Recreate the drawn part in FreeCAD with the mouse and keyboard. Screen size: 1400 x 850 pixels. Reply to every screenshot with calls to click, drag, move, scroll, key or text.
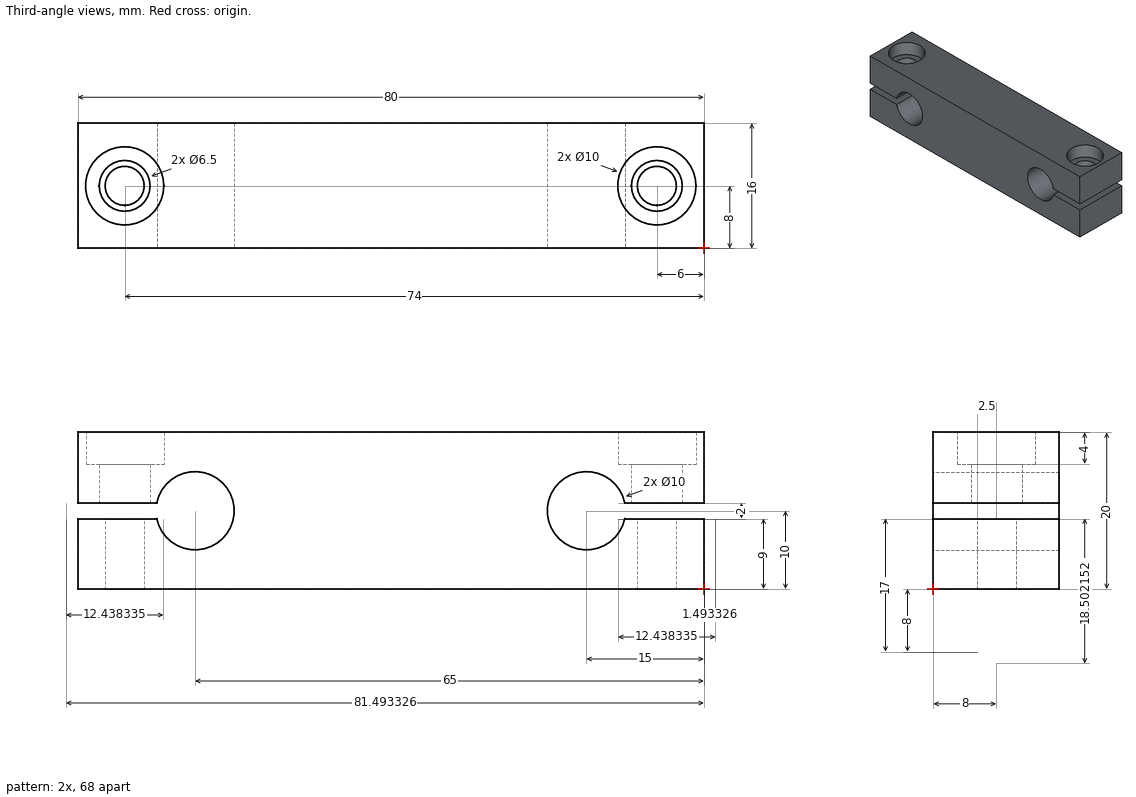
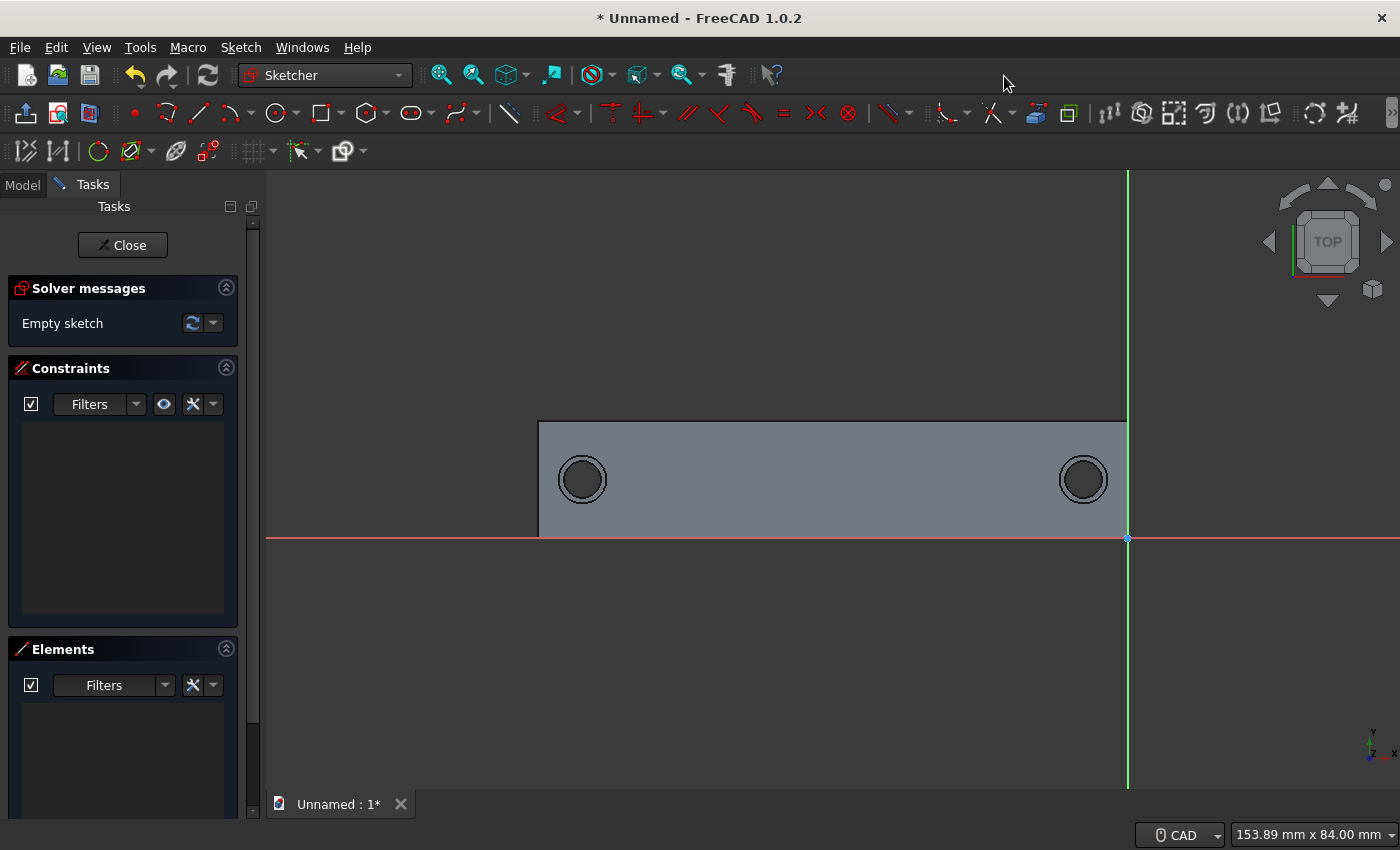
click(276, 114)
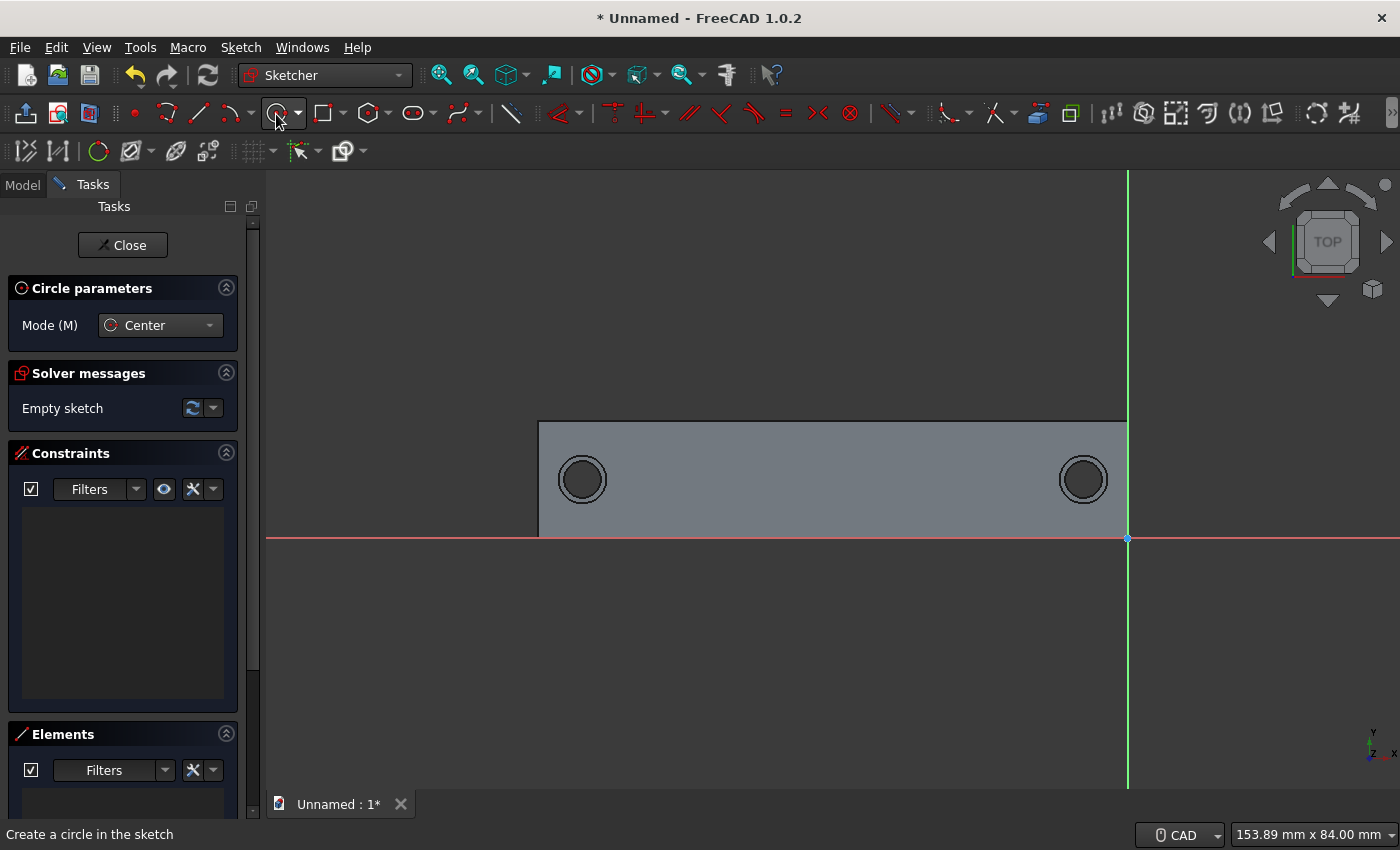
click(1084, 480)
click(1110, 453)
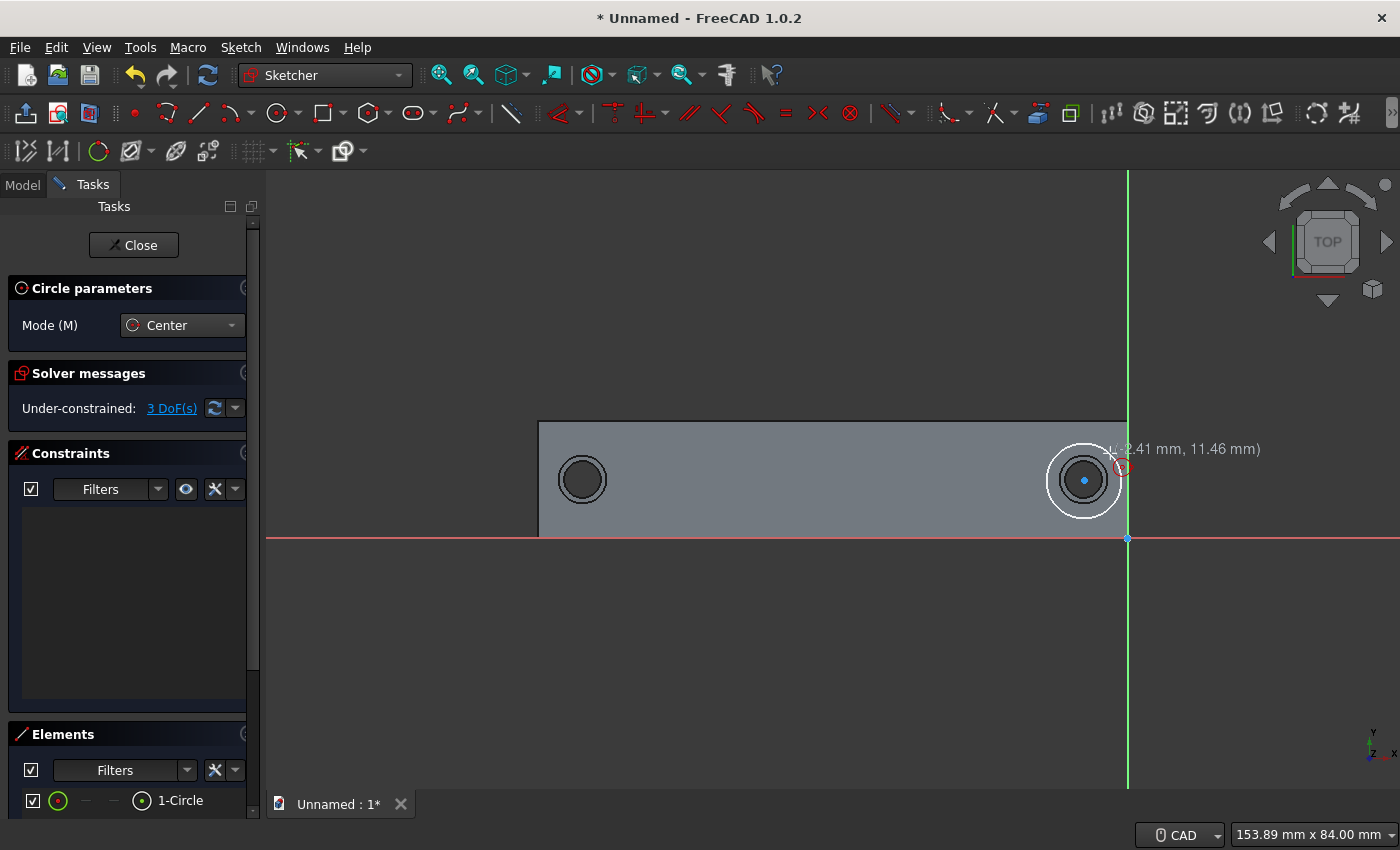
click(582, 480)
click(609, 453)
key(Escape)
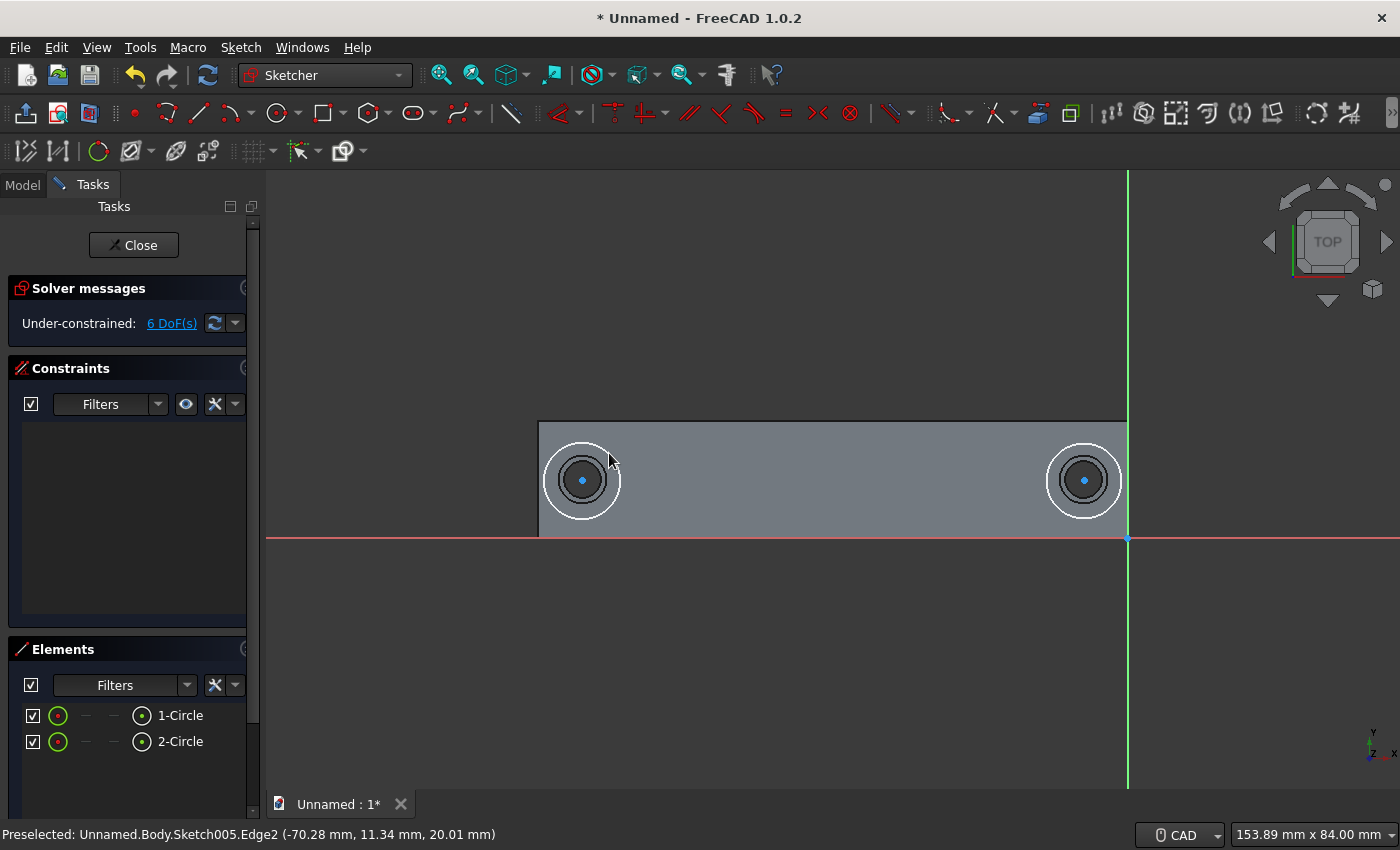
click(1110, 454)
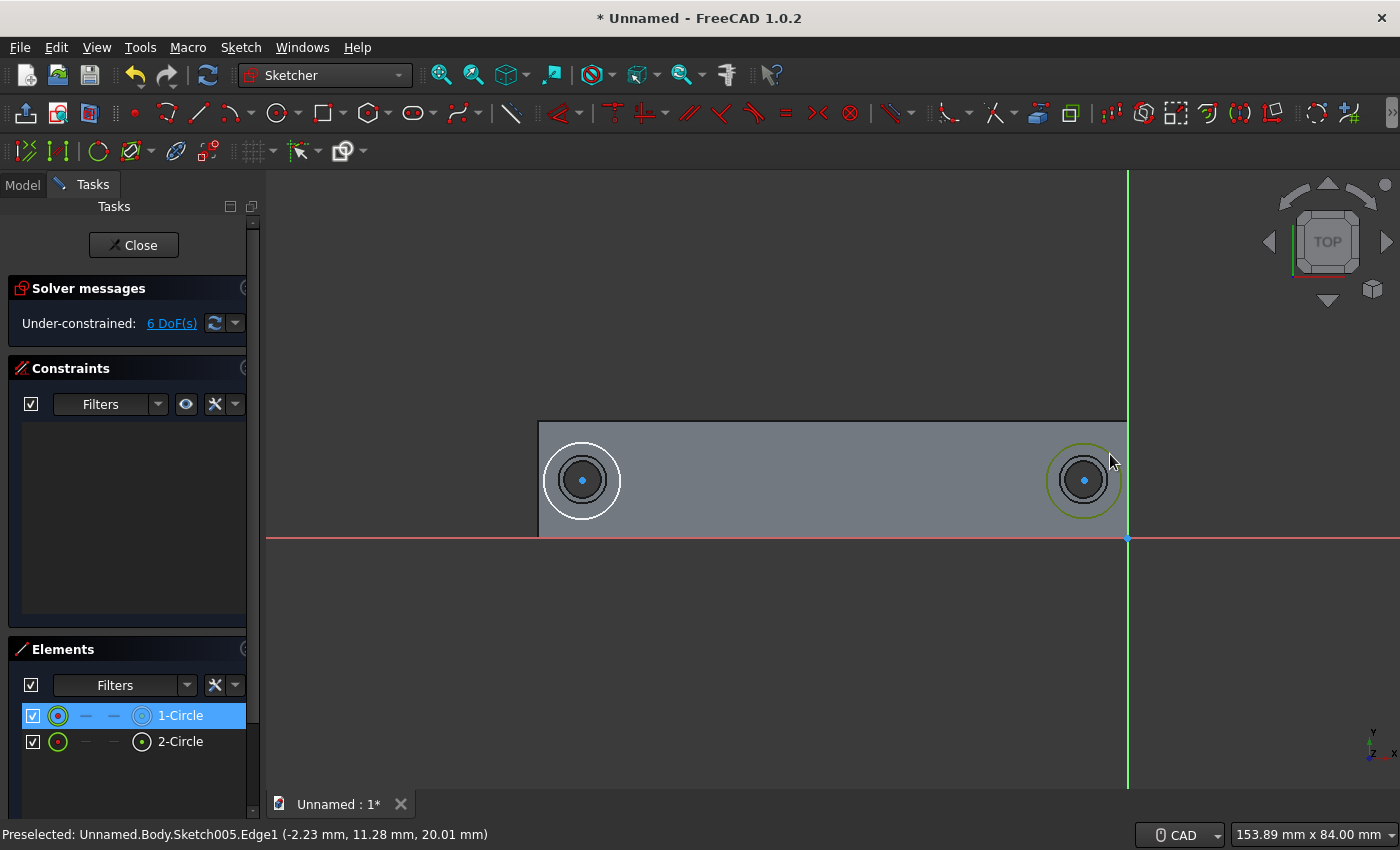
click(609, 454)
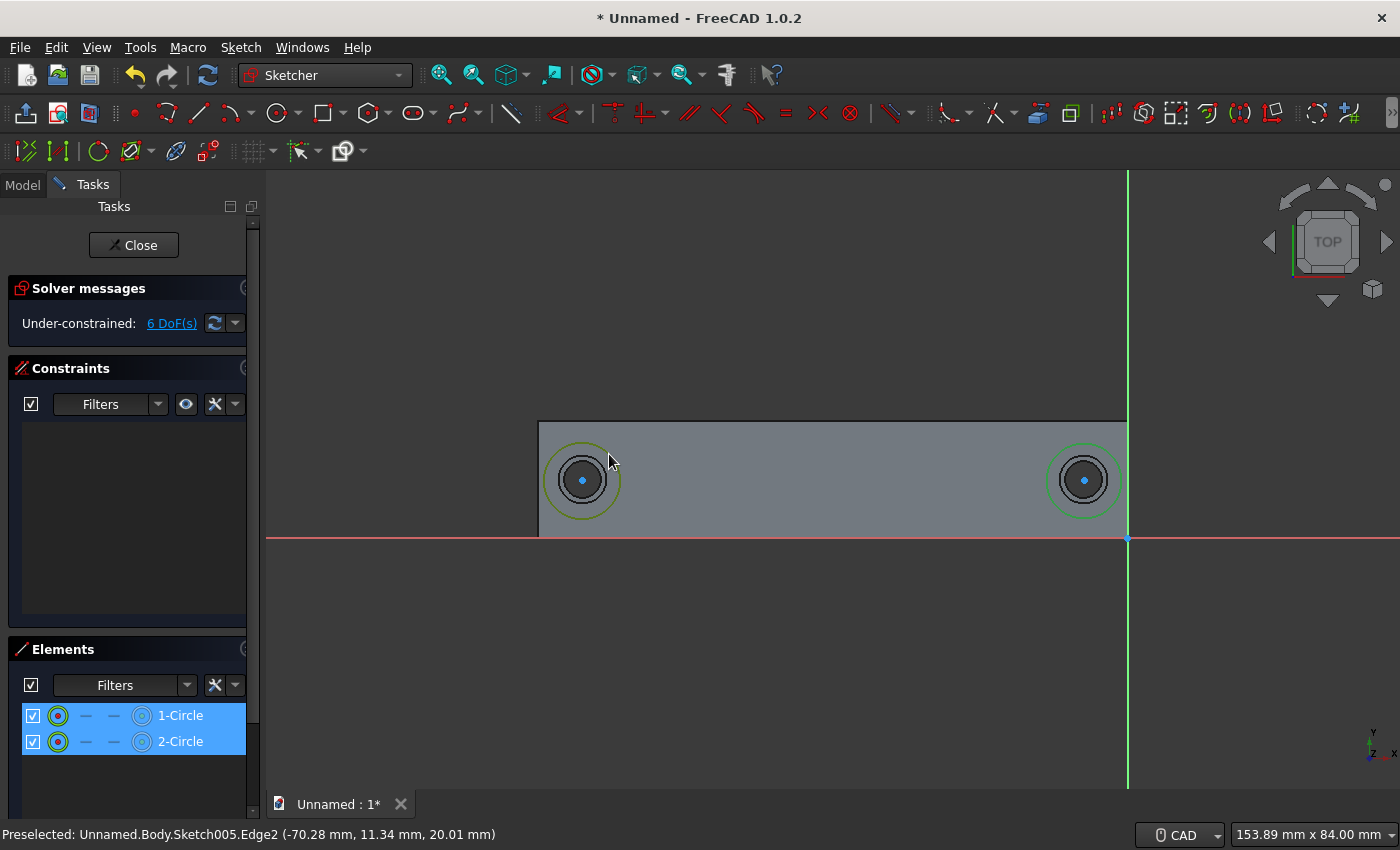
click(786, 114)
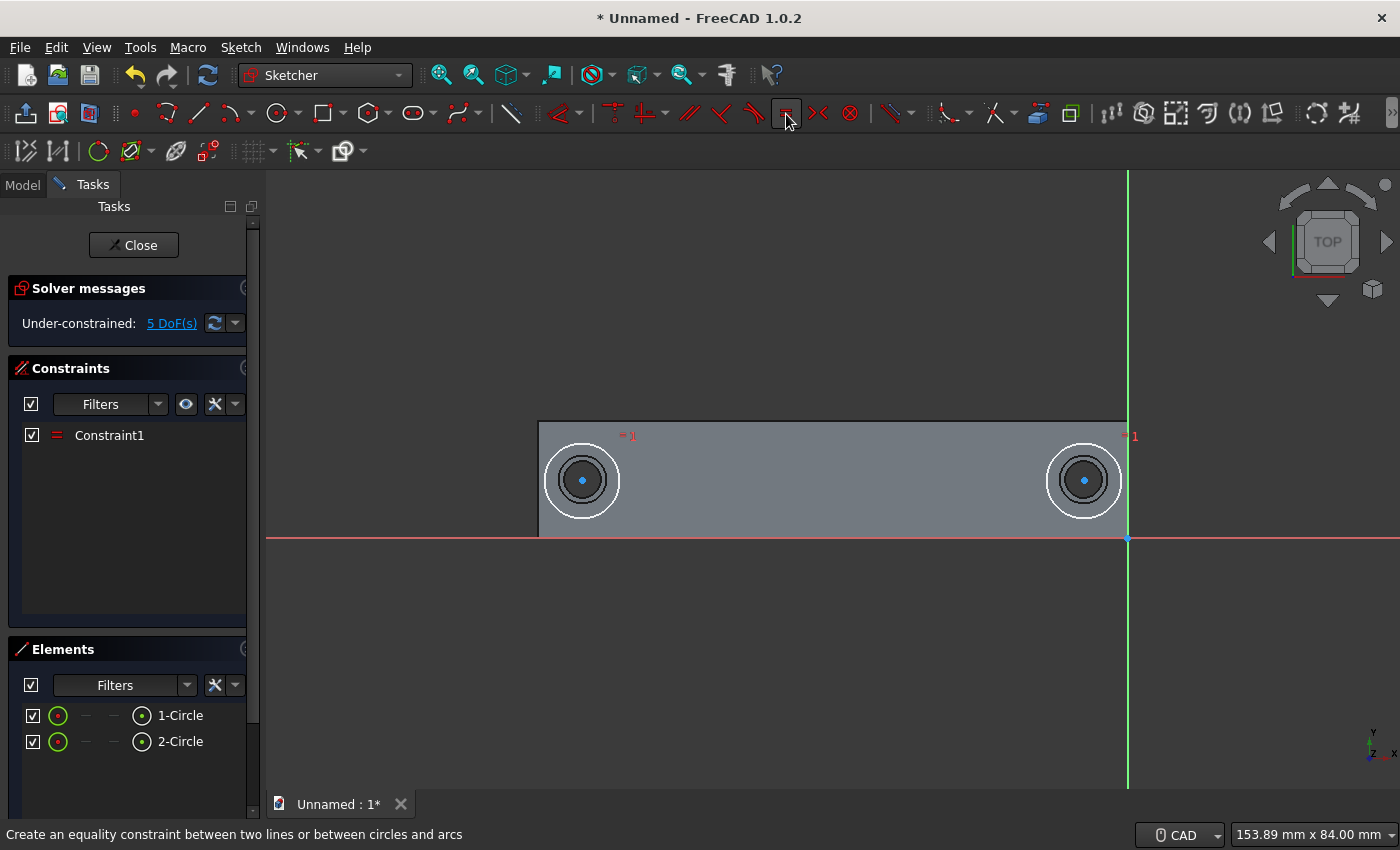
click(558, 114)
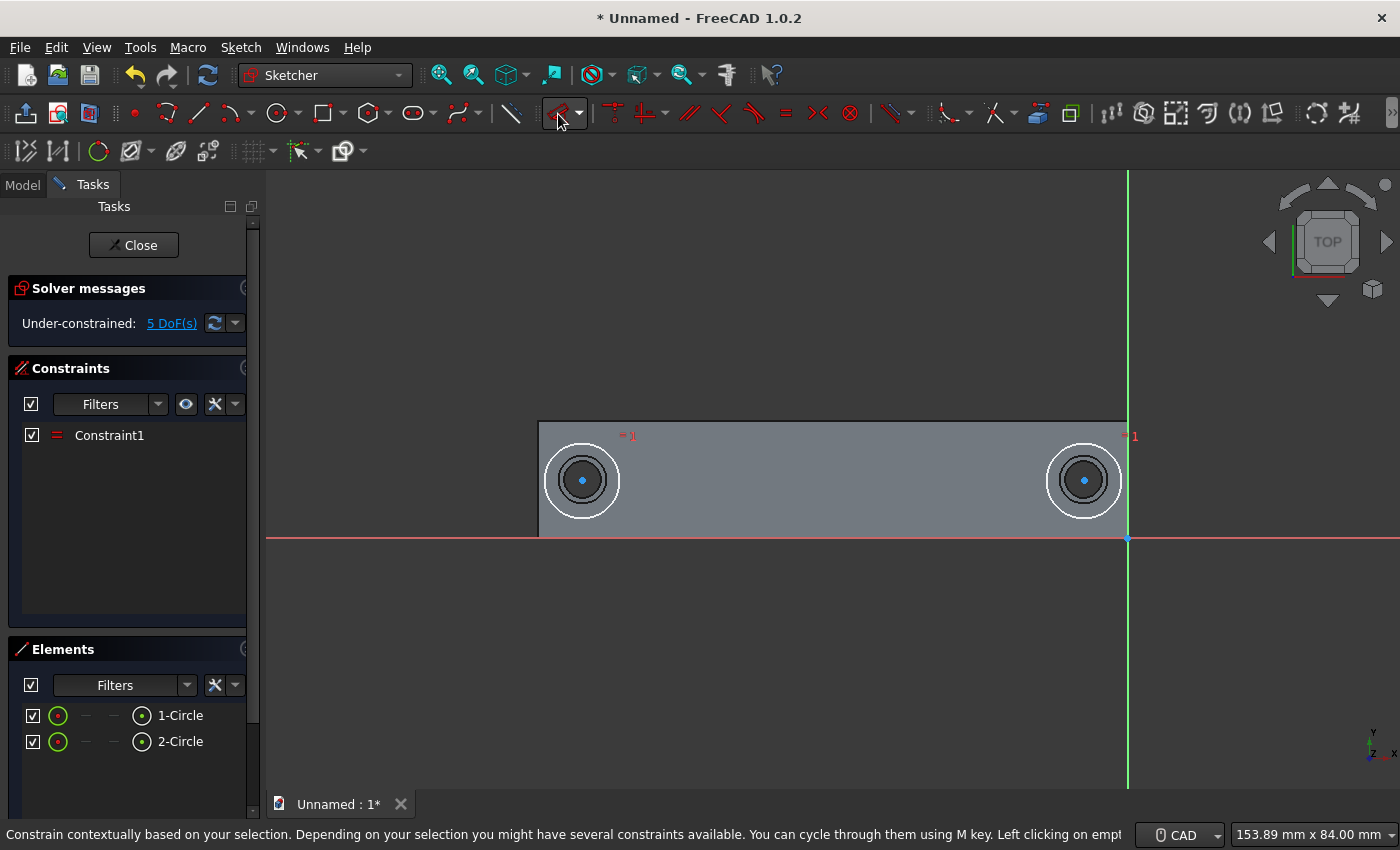
click(1110, 454)
click(1150, 460)